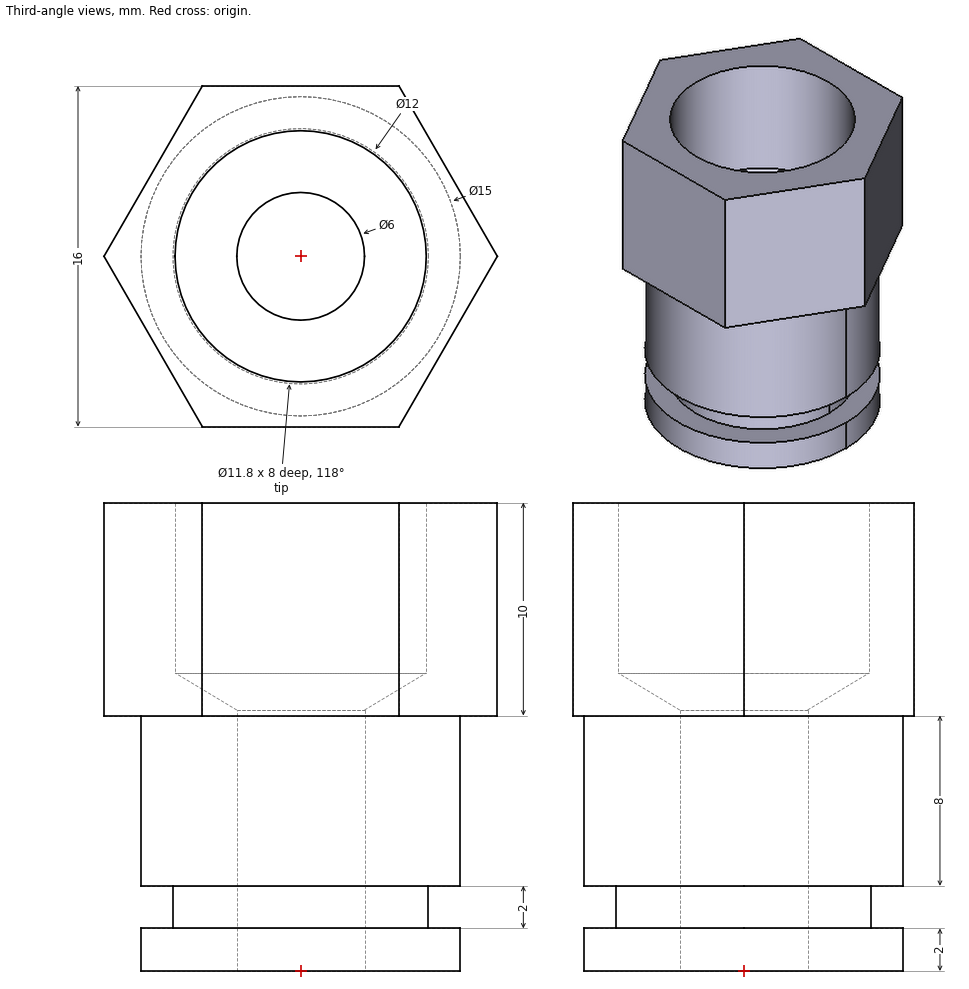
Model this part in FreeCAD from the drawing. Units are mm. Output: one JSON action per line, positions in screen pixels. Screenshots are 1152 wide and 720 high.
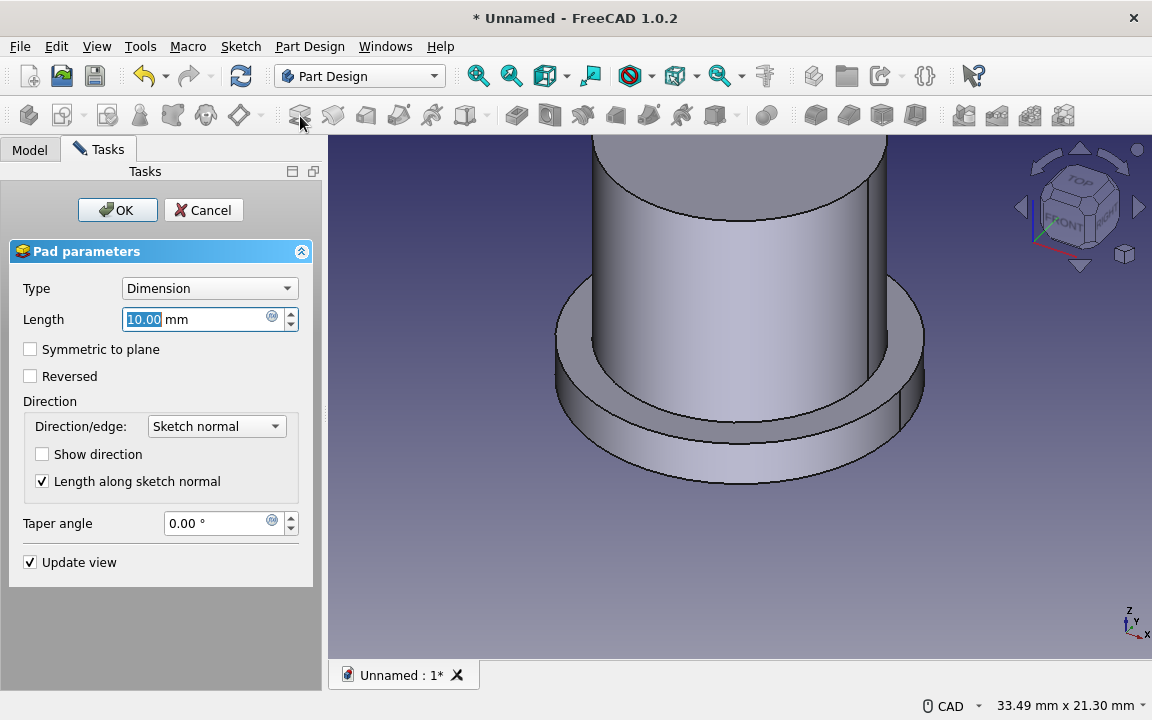
{"action": "type", "text": "2"}
{"action": "key", "text": "Tab"}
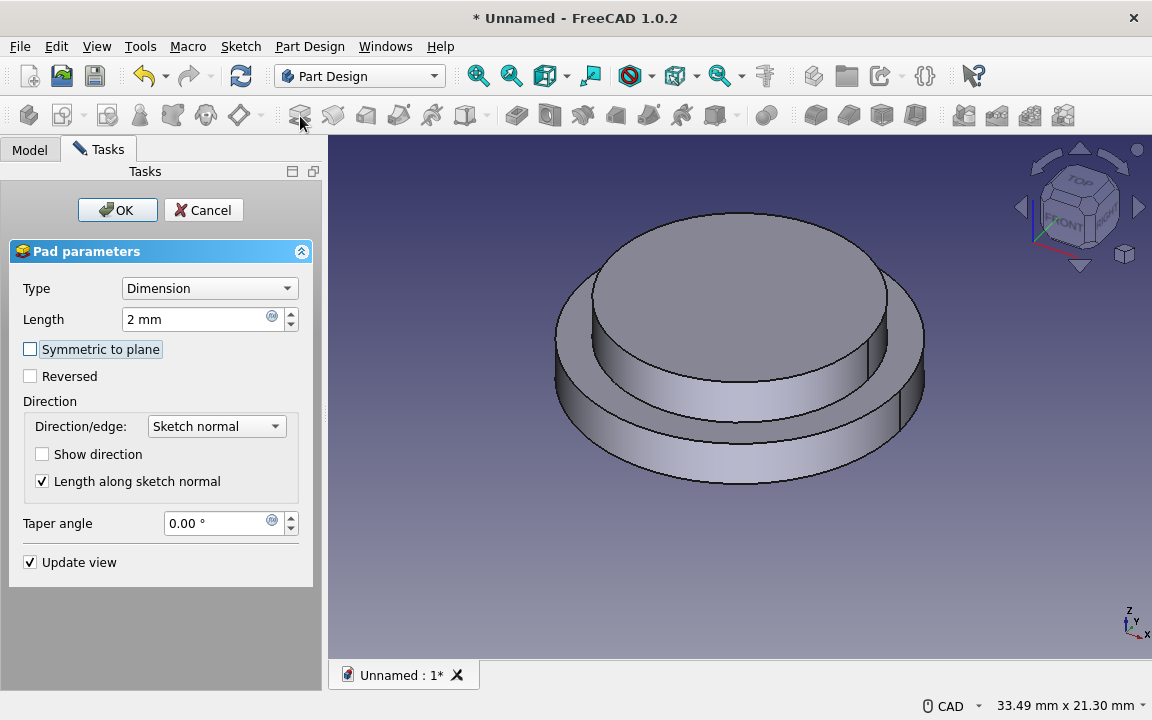
{"action": "left_click", "coordinate": [118, 210]}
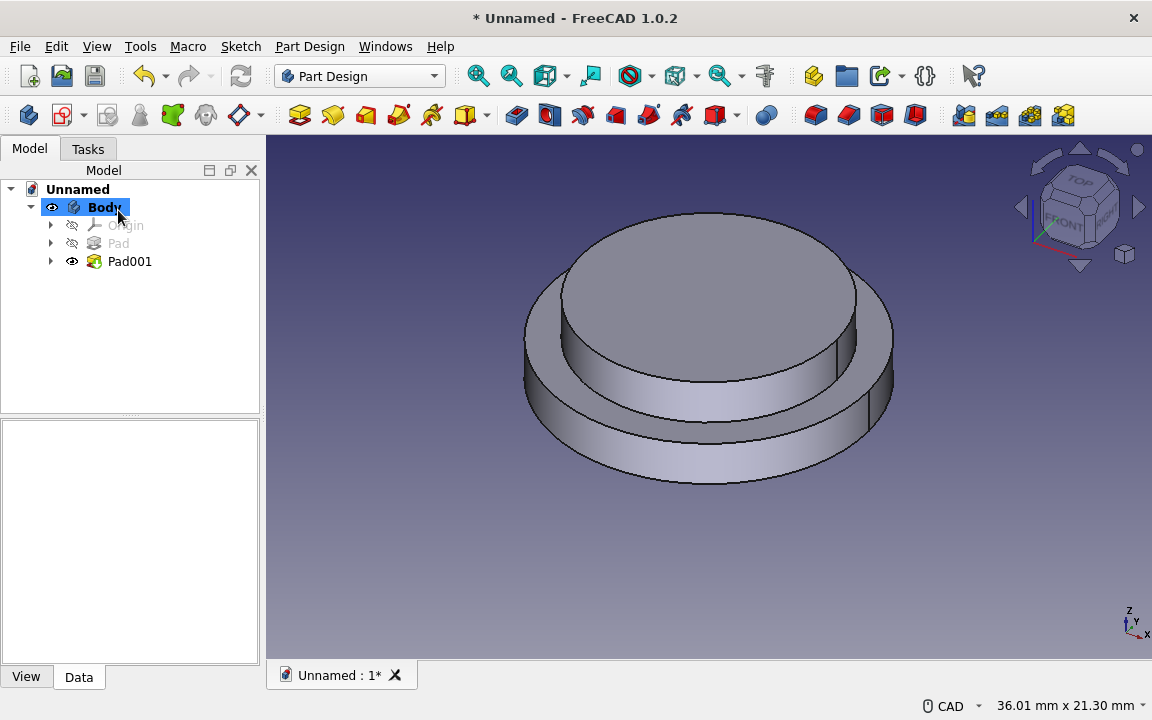
{"action": "left_click", "coordinate": [709, 297]}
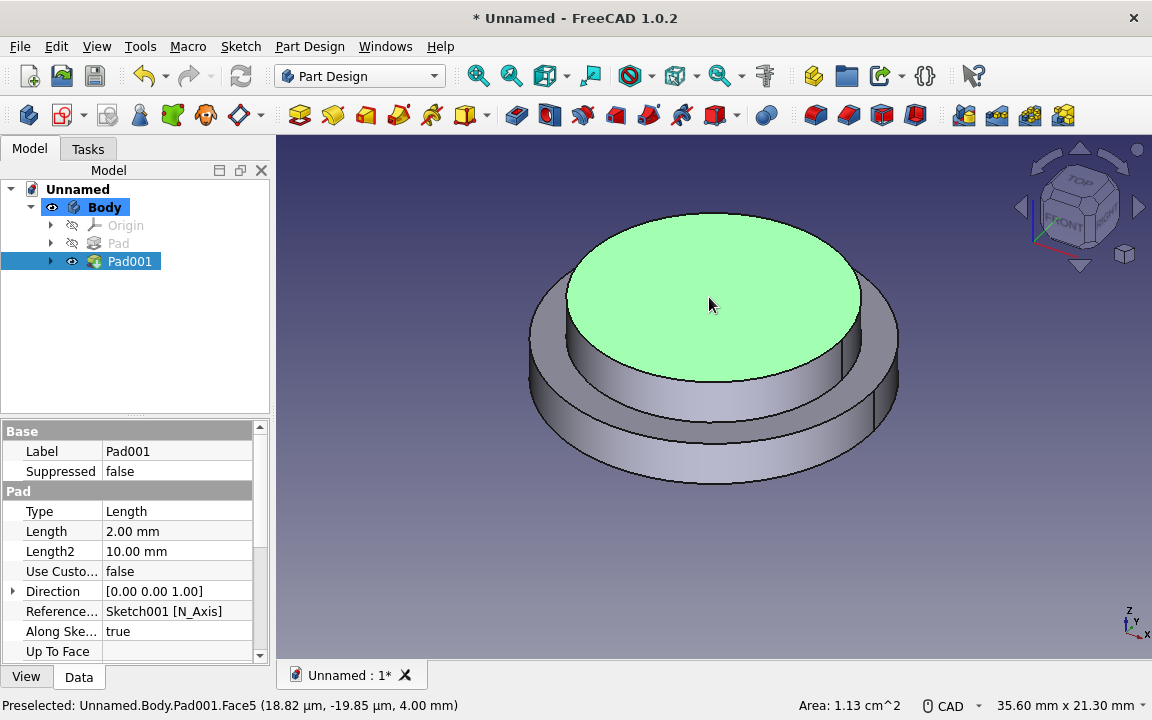
{"action": "left_click", "coordinate": [62, 116]}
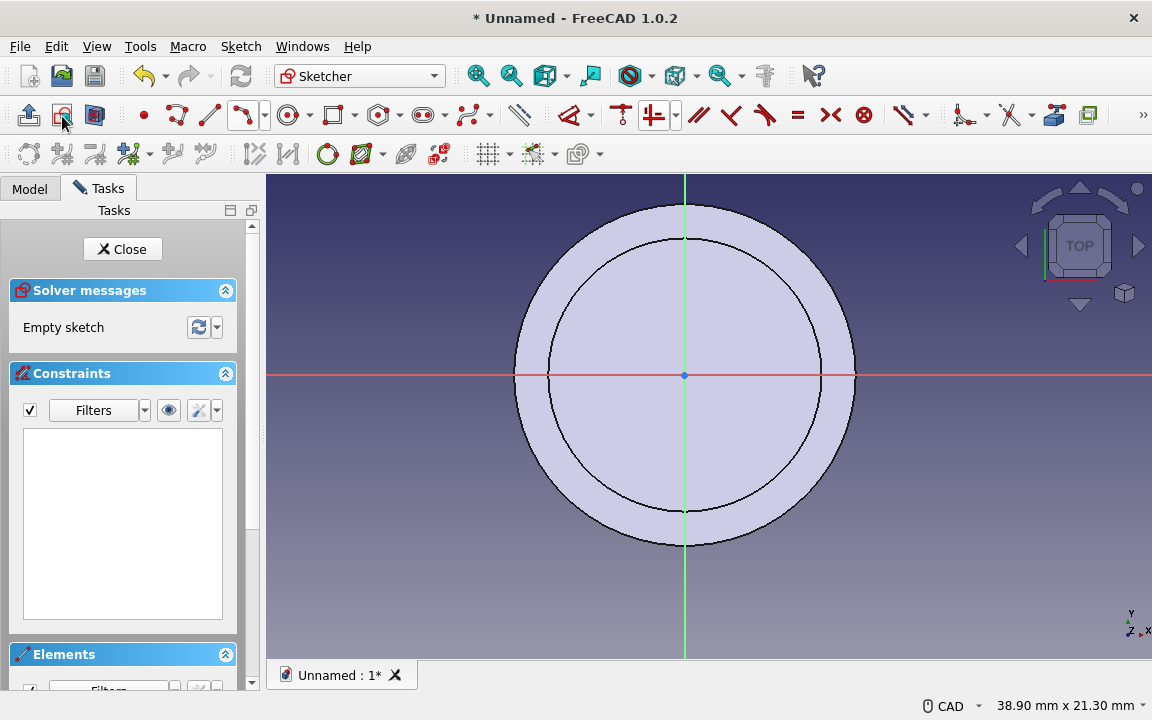
{"action": "scroll", "coordinate": [440, 604], "scroll_direction": "down", "scroll_amount": 1}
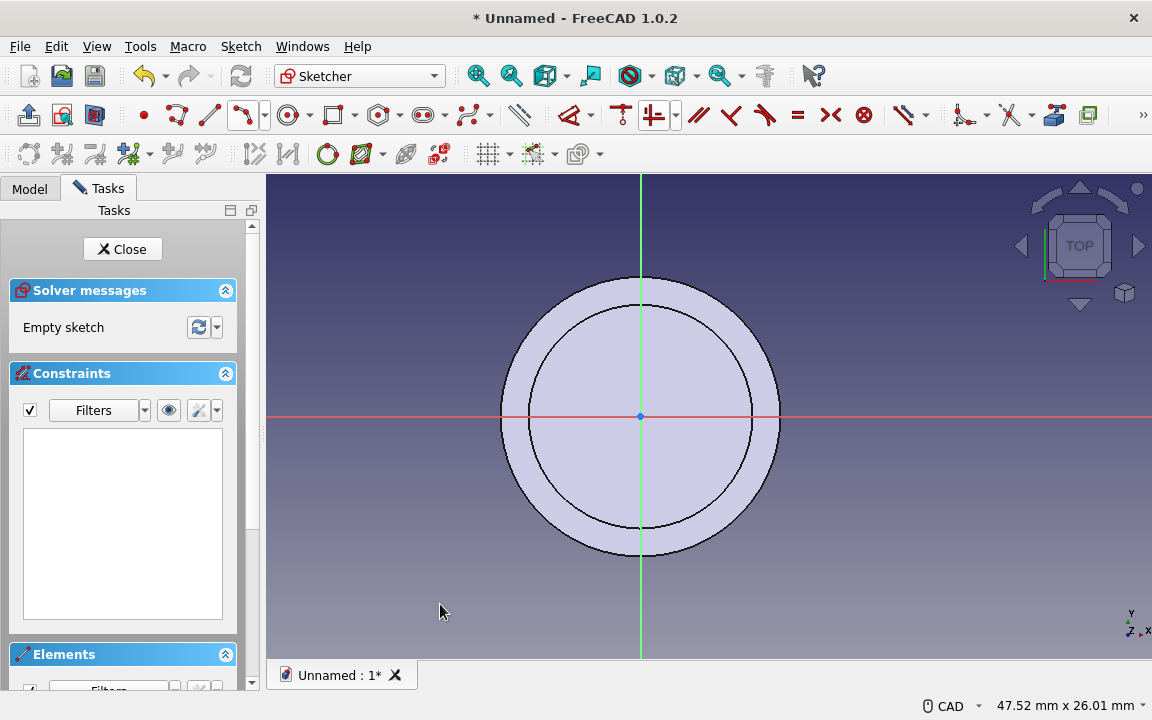
{"action": "left_click", "coordinate": [288, 116]}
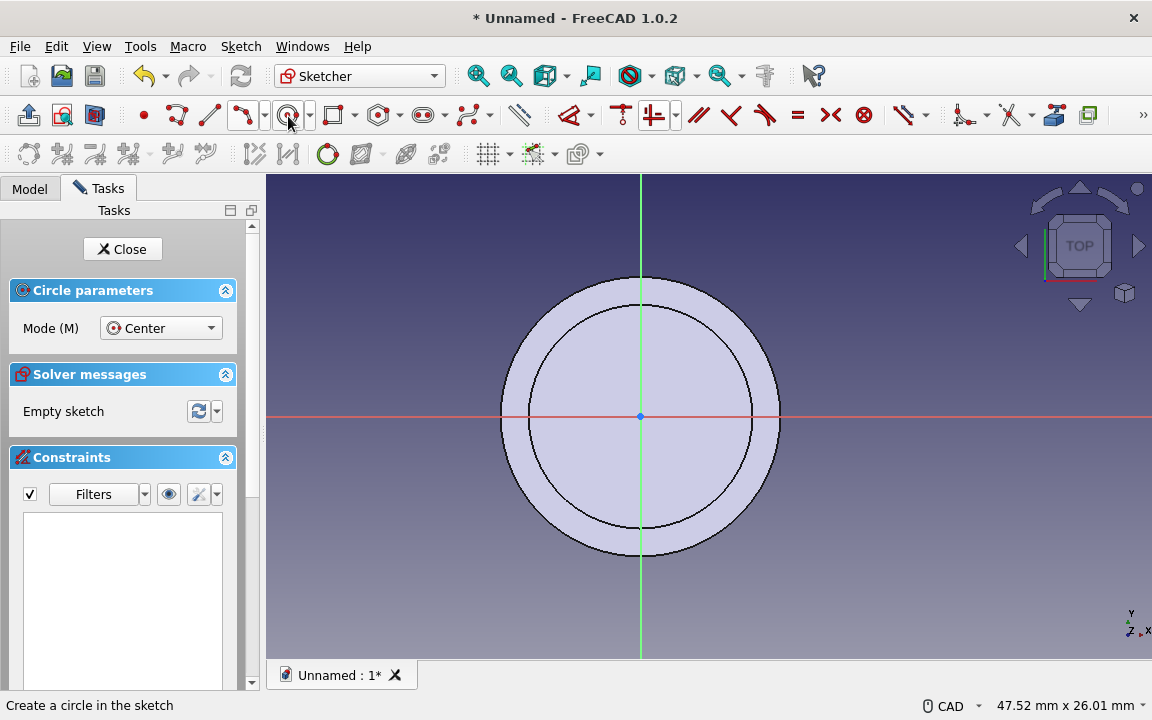
{"action": "left_click", "coordinate": [641, 417]}
{"action": "left_click", "coordinate": [739, 318]}
{"action": "key", "text": "Escape"}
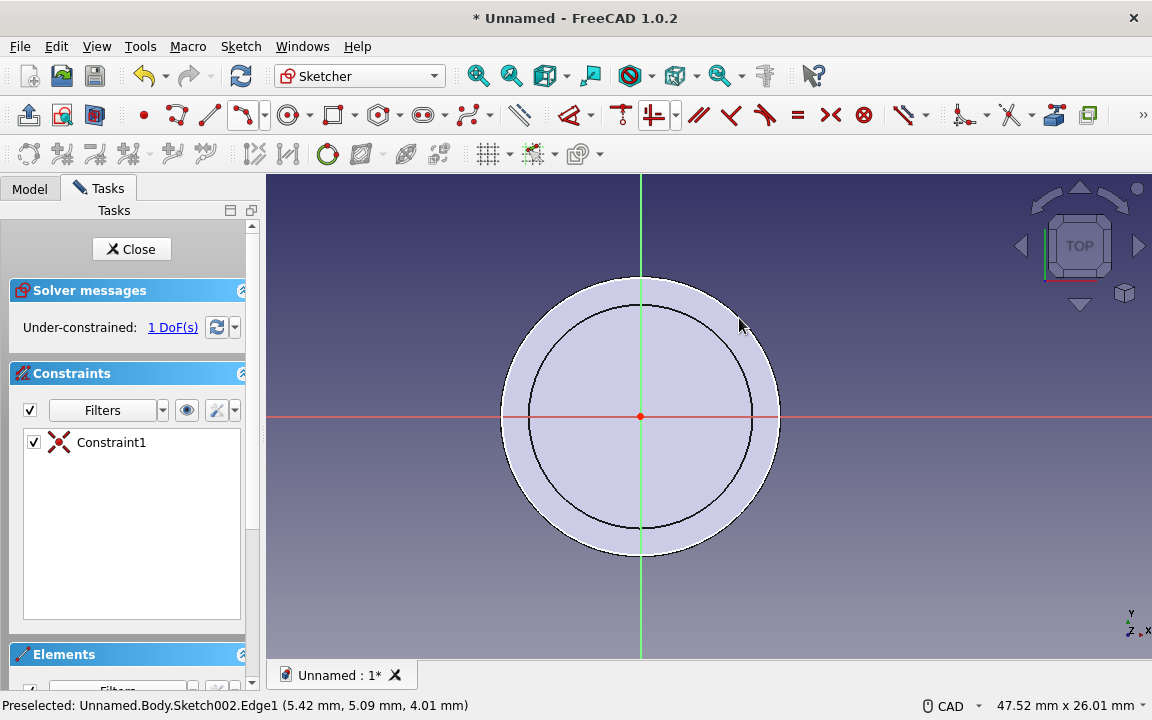
{"action": "key", "text": "d"}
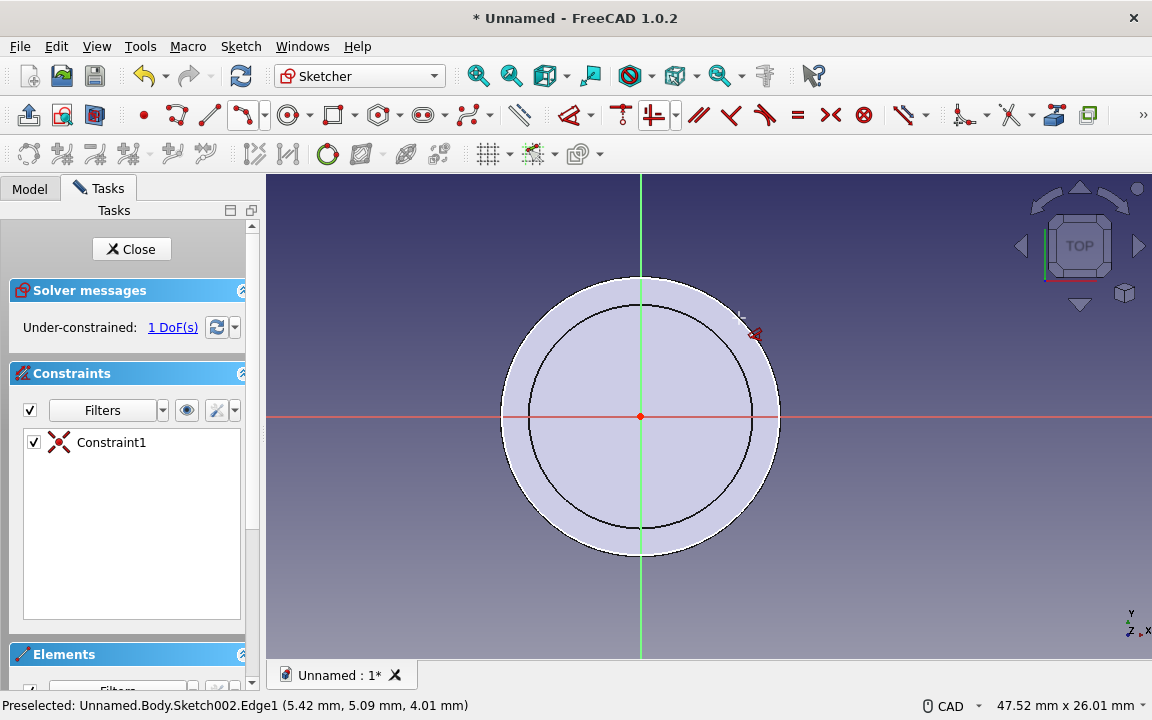
{"action": "left_click", "coordinate": [738, 318]}
{"action": "left_click", "coordinate": [760, 295]}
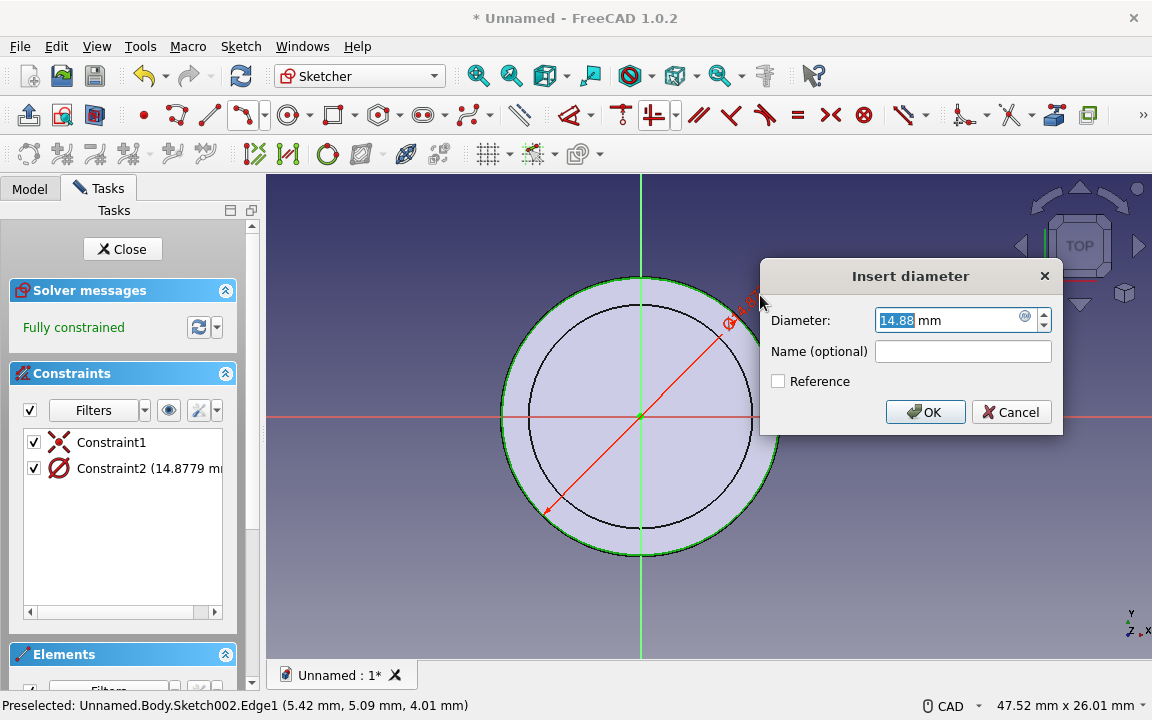
{"action": "type", "text": "15"}
{"action": "key", "text": "Return"}
{"action": "key", "text": "Escape"}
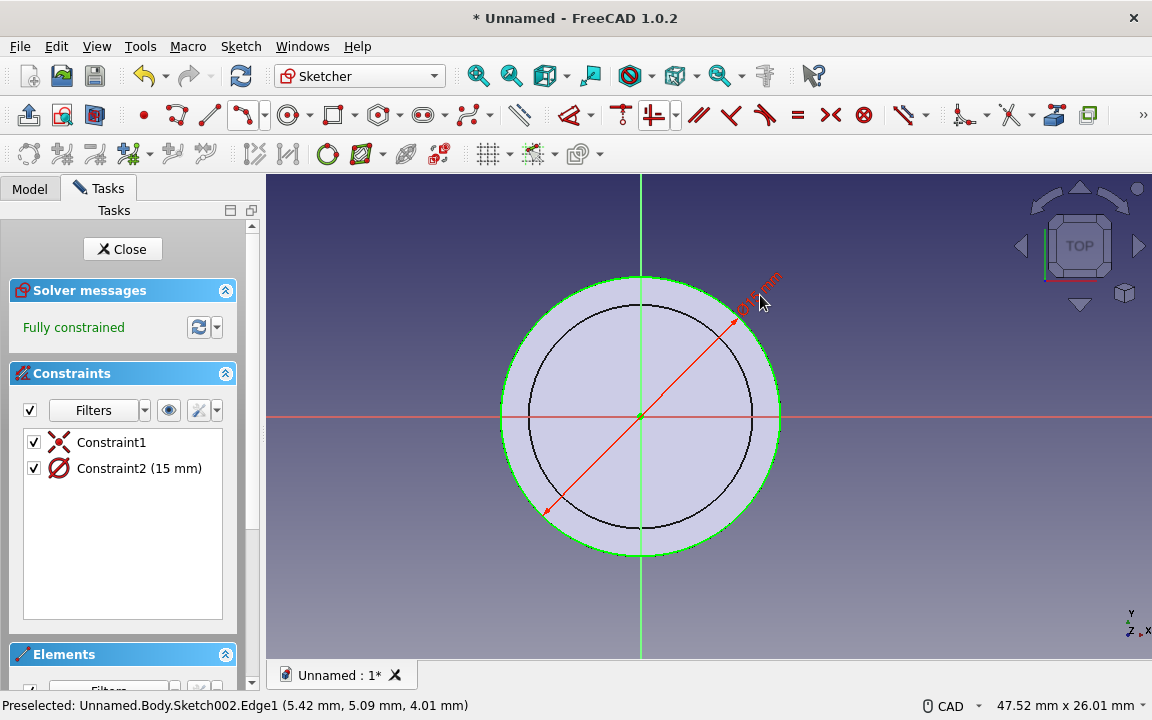
{"action": "left_click", "coordinate": [123, 249]}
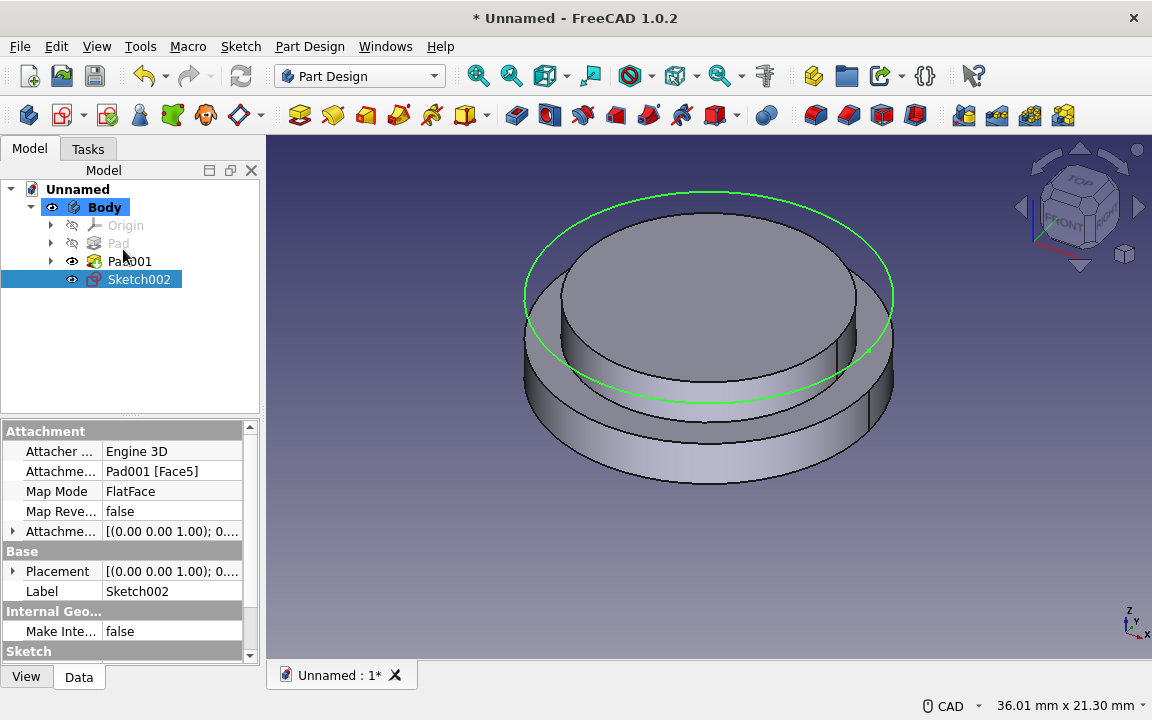
{"action": "left_click", "coordinate": [300, 116]}